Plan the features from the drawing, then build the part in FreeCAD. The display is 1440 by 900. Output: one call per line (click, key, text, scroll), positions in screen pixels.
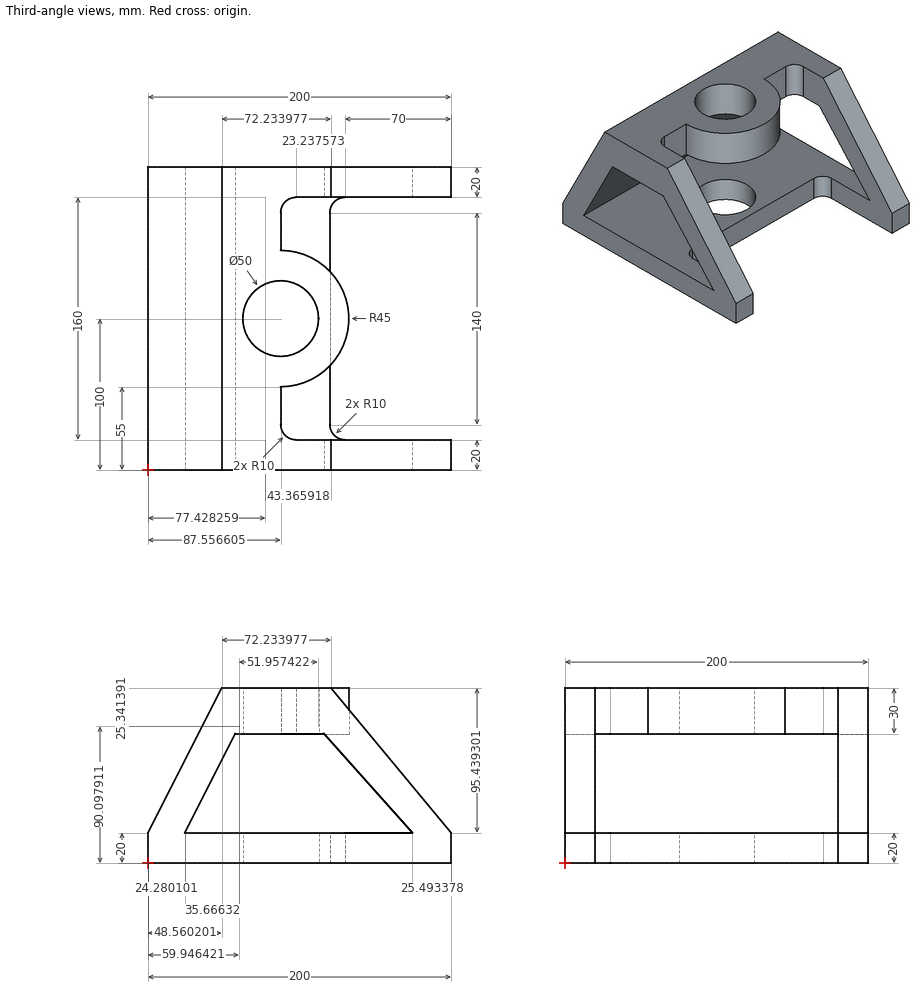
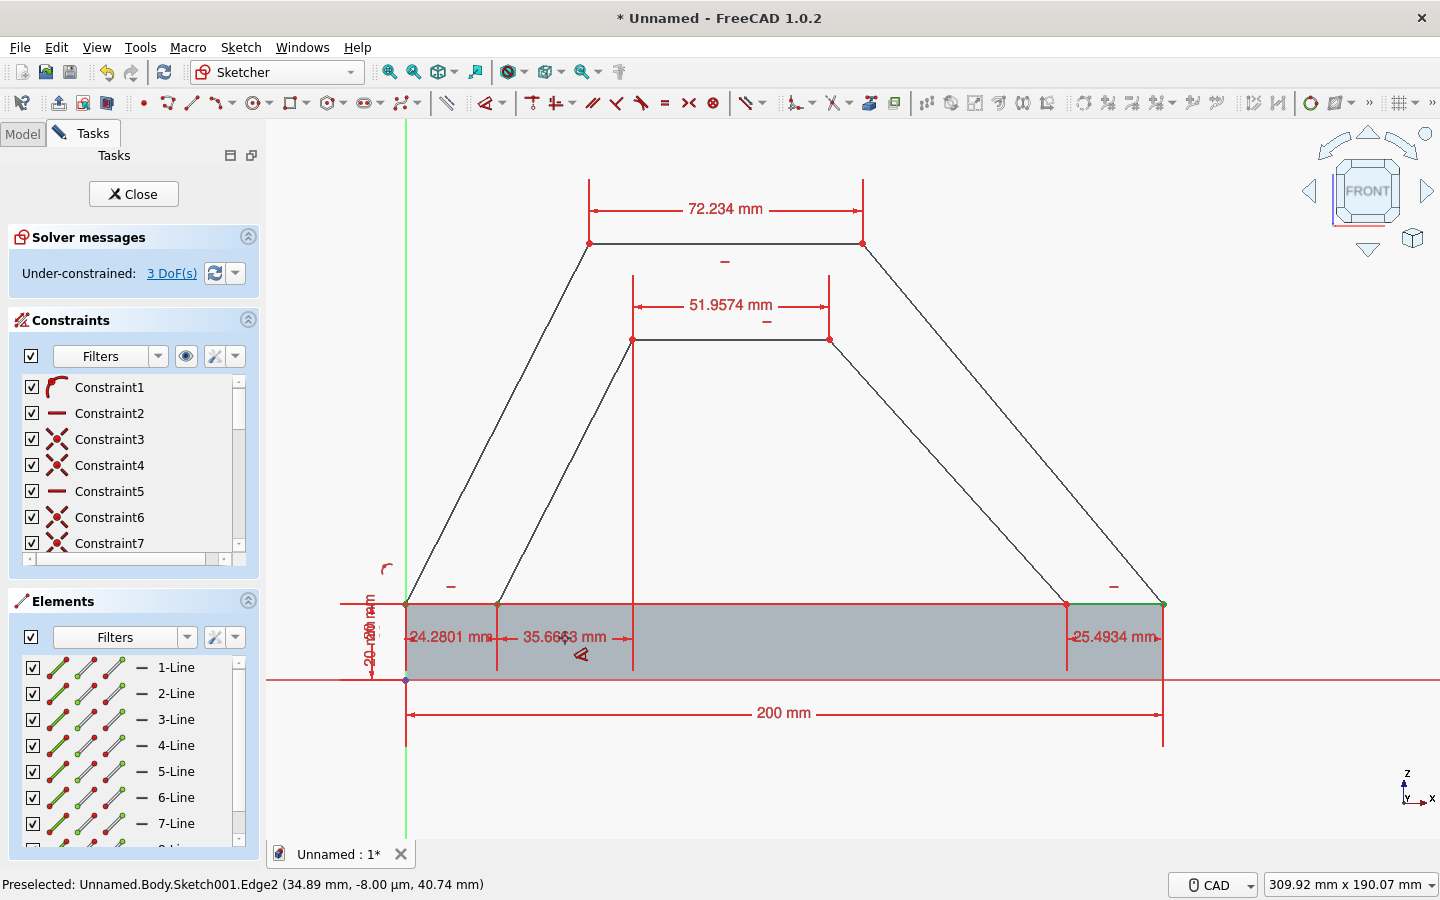
click(633, 340)
click(372, 510)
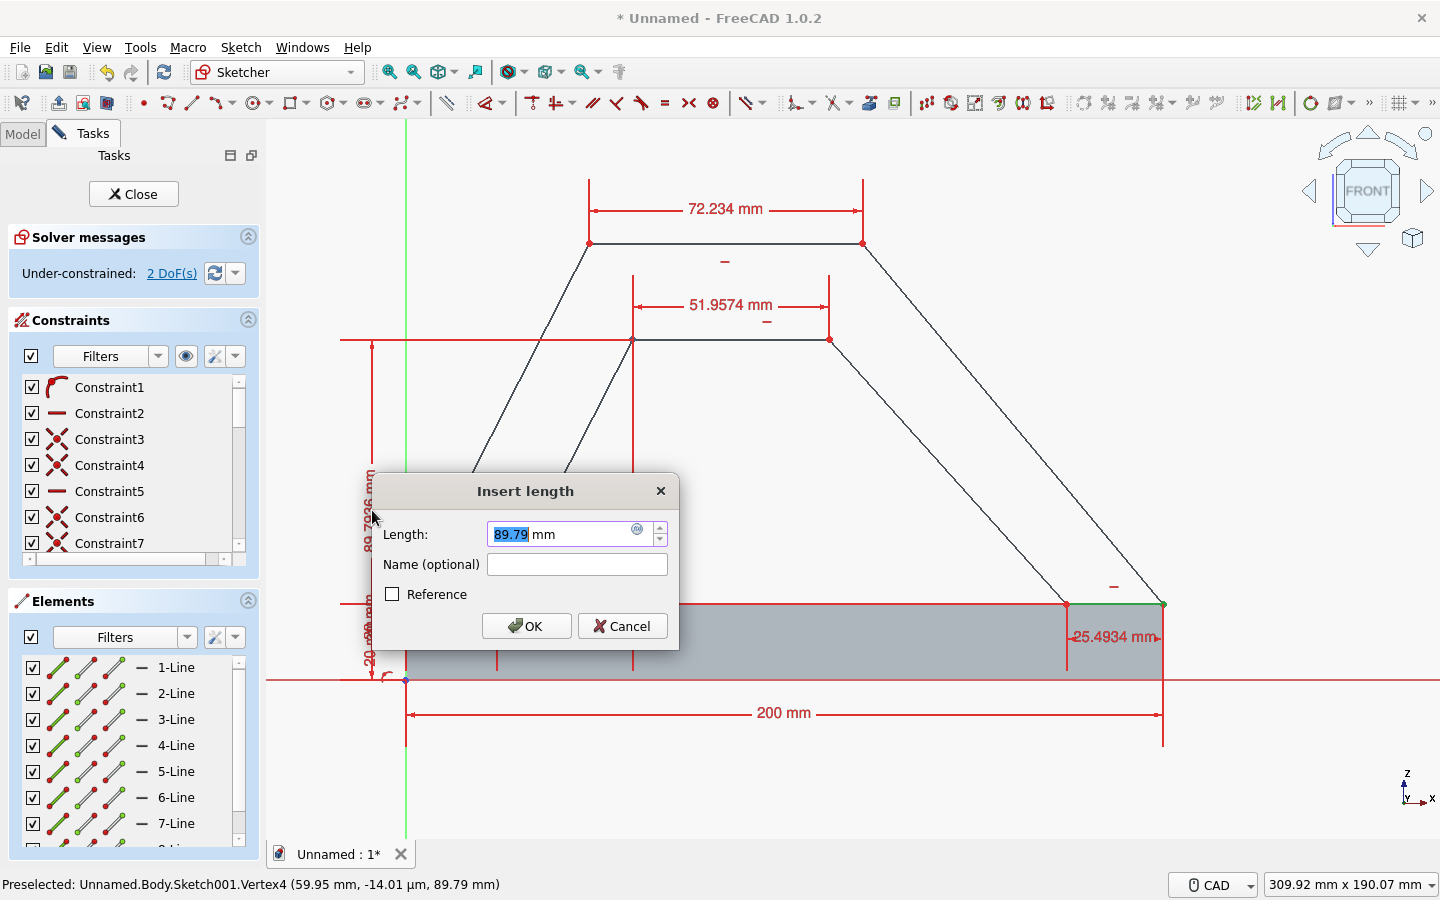
text(90.097911)
key(Return)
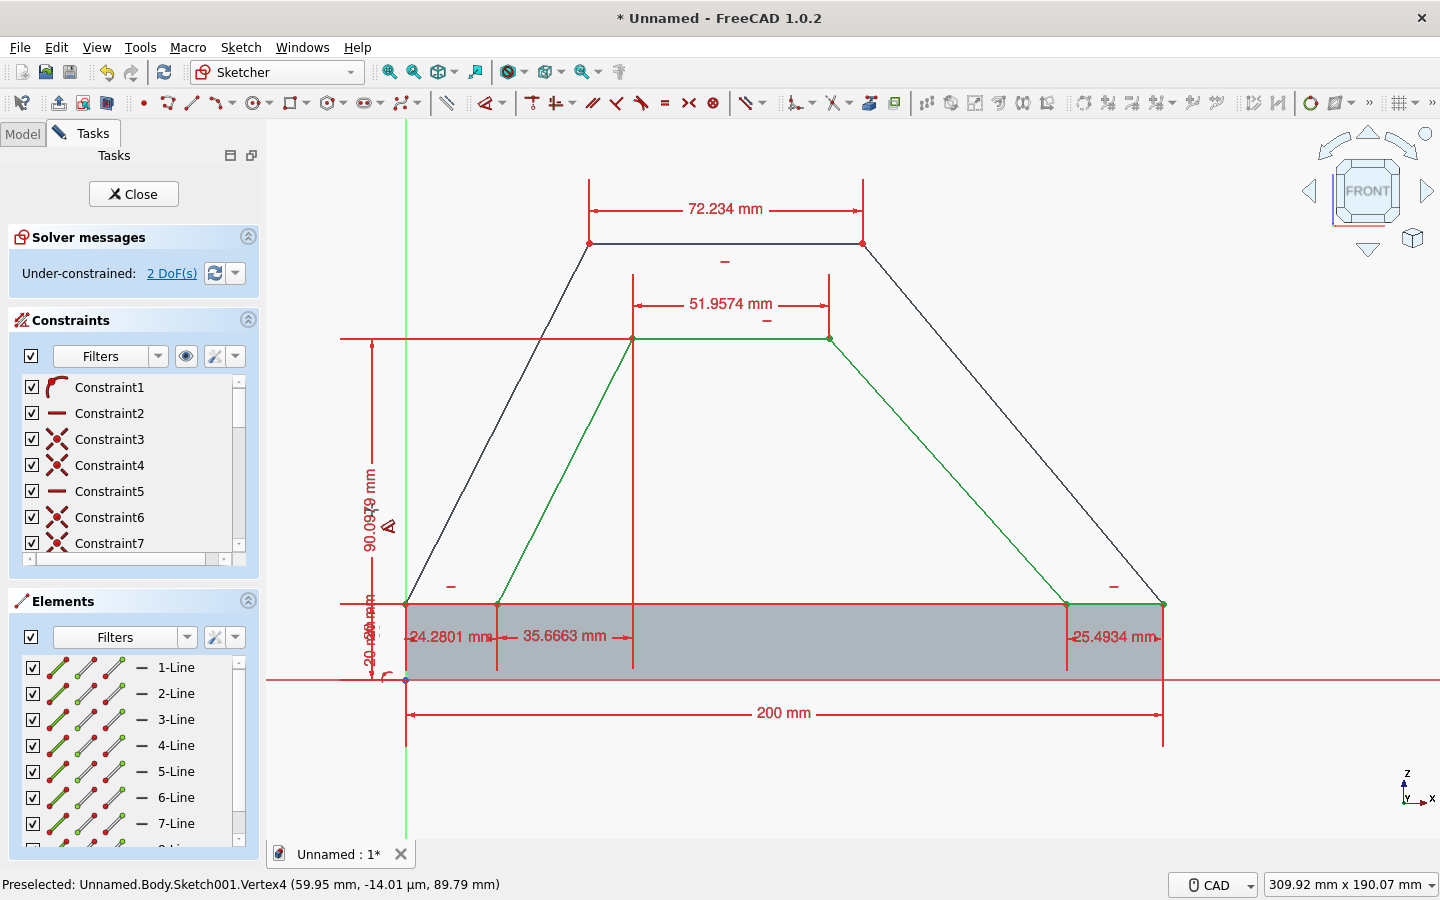
click(589, 244)
click(497, 714)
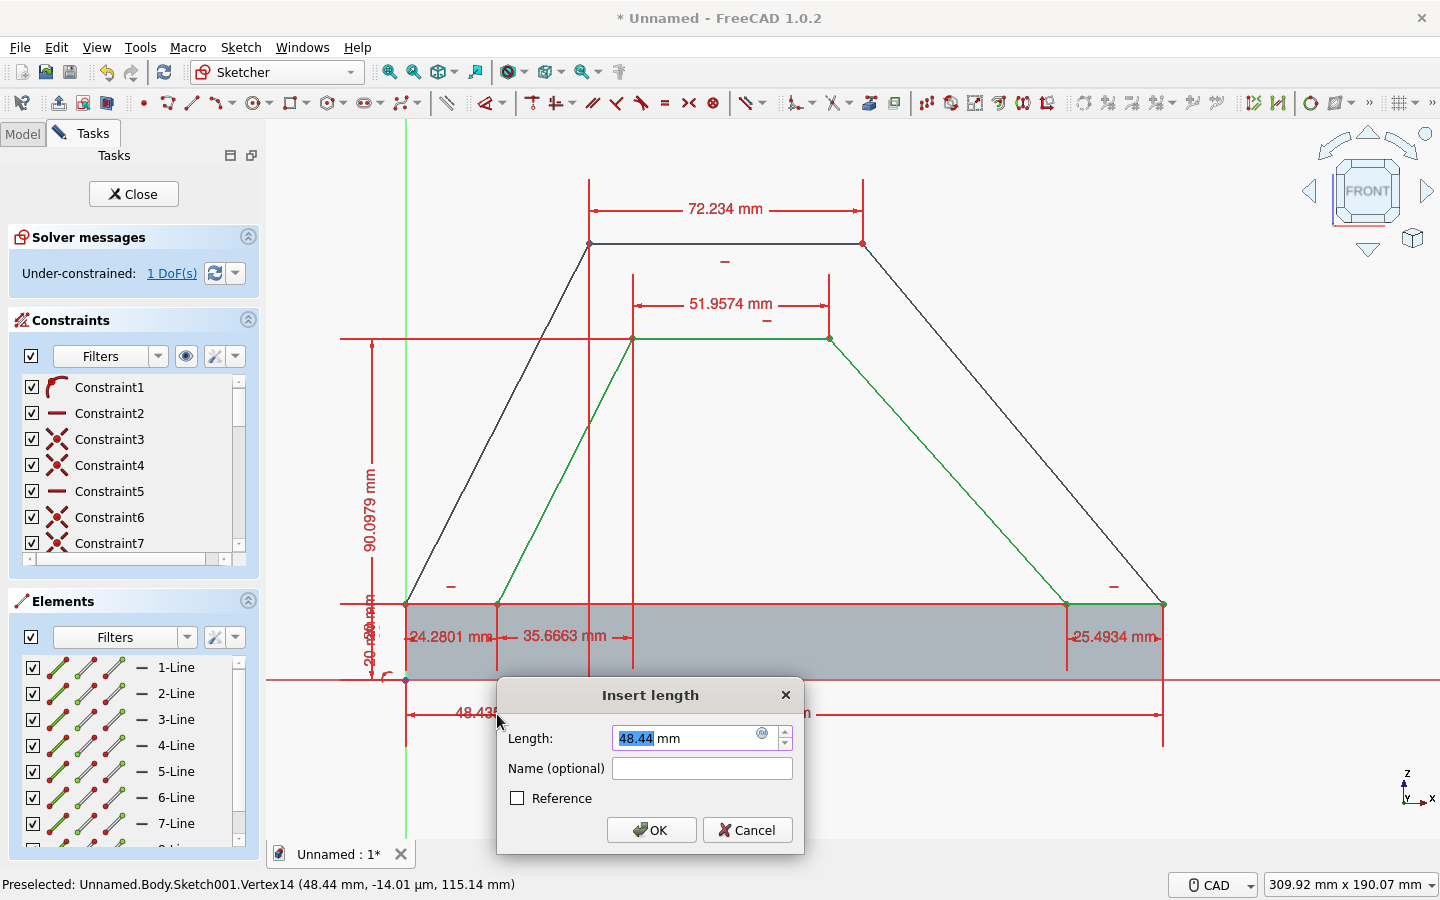
text(48.560201)
key(Return)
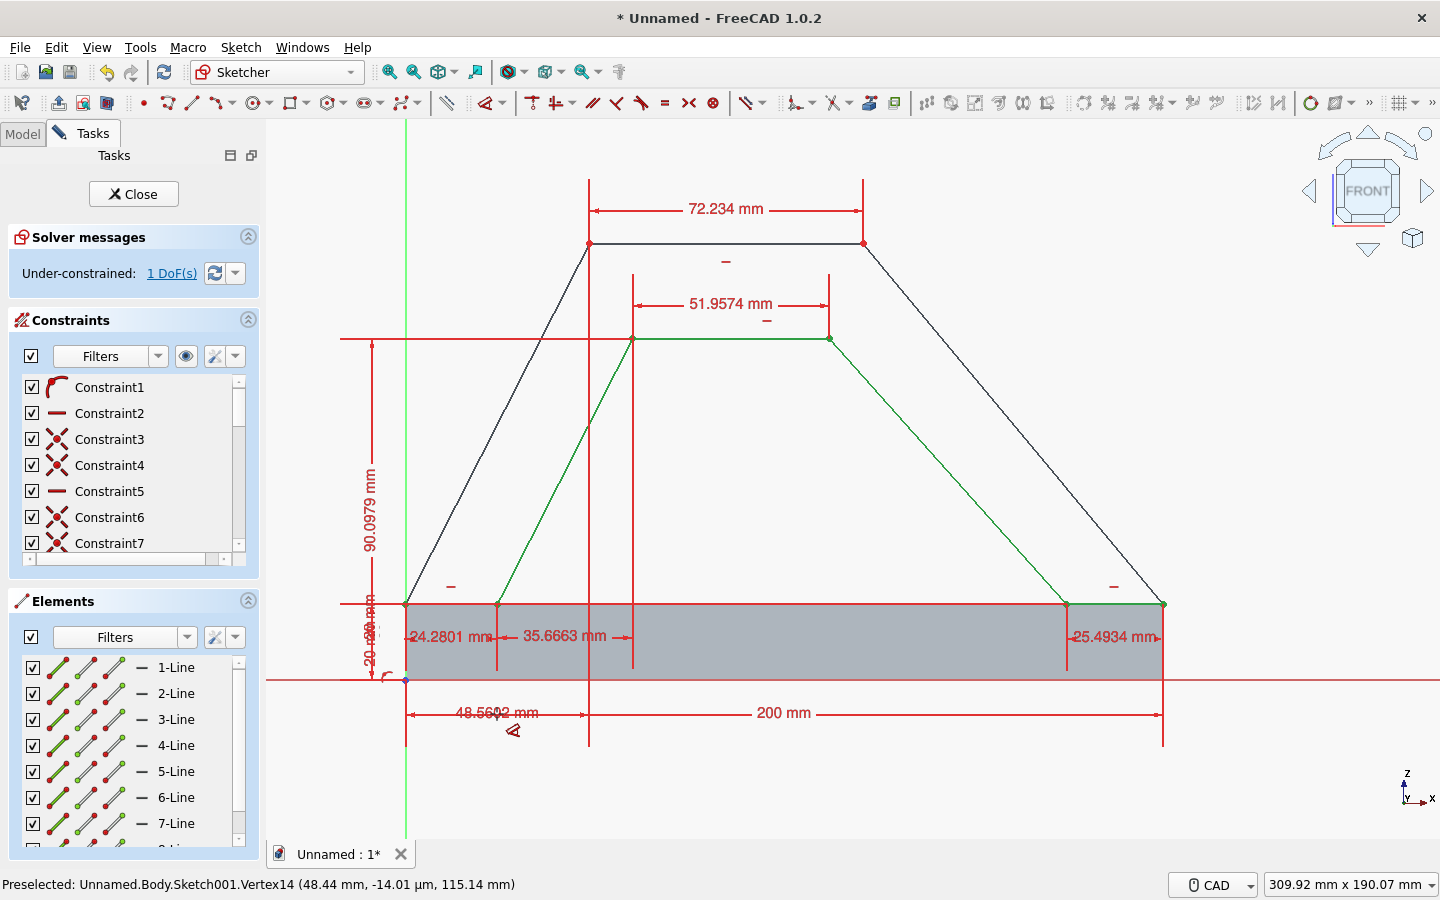
click(1073, 496)
click(1197, 424)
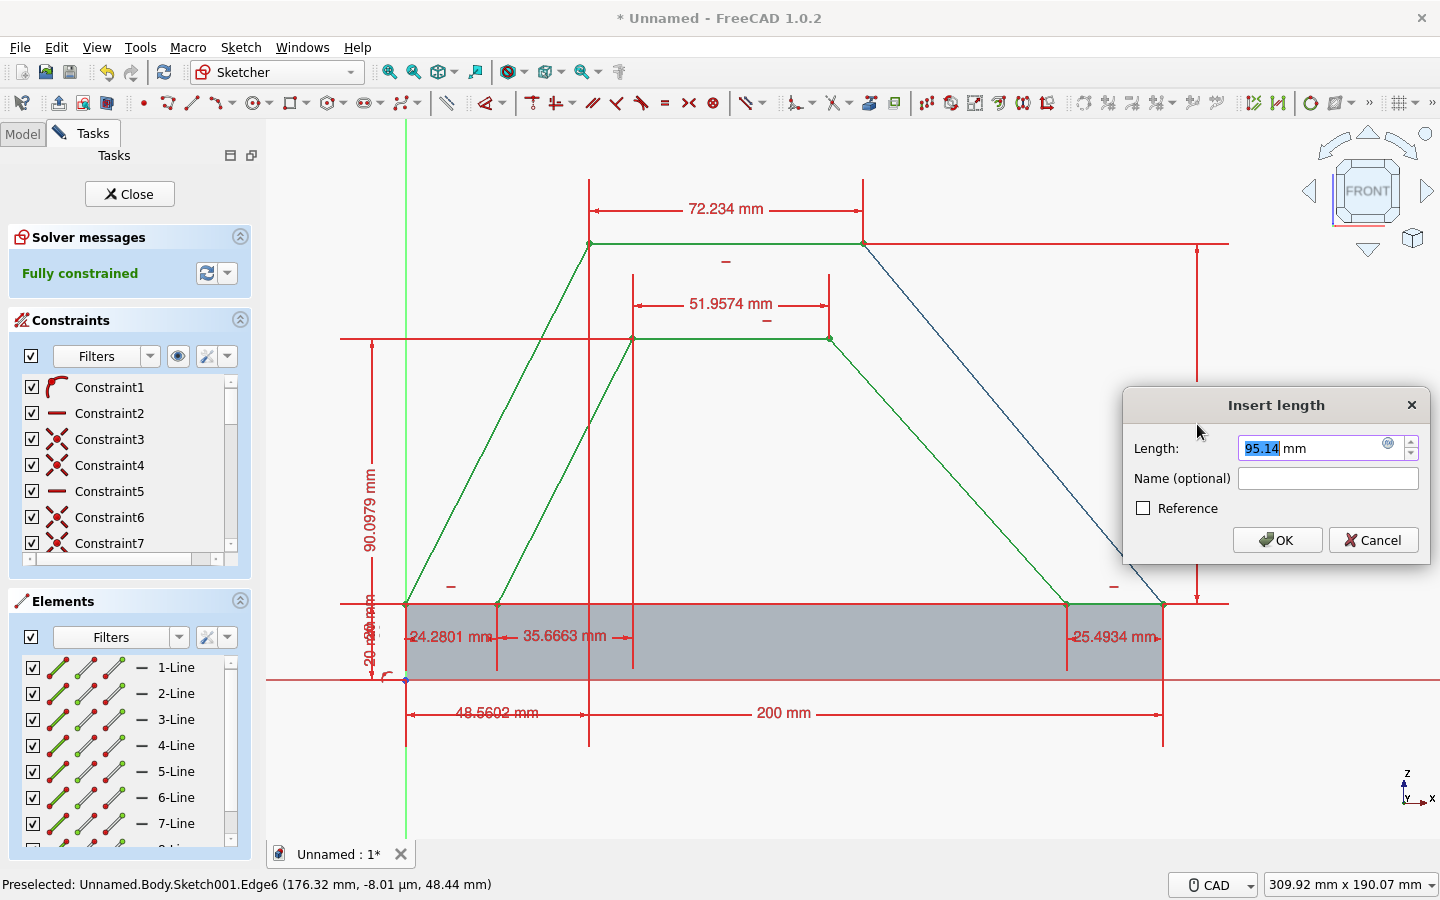
text(95.439301)
key(Return)
key(Escape)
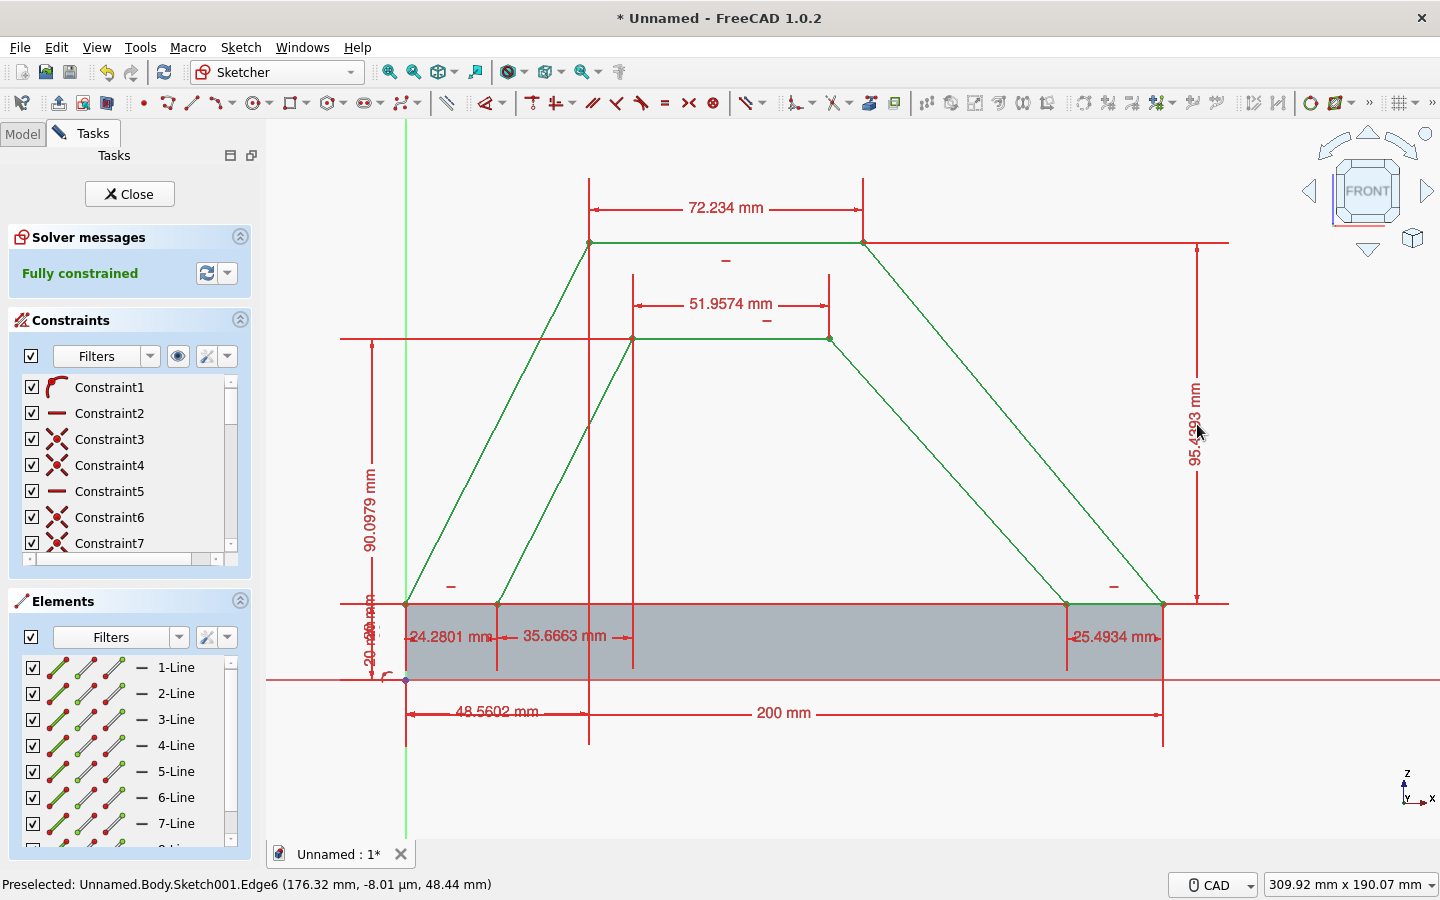
click(130, 194)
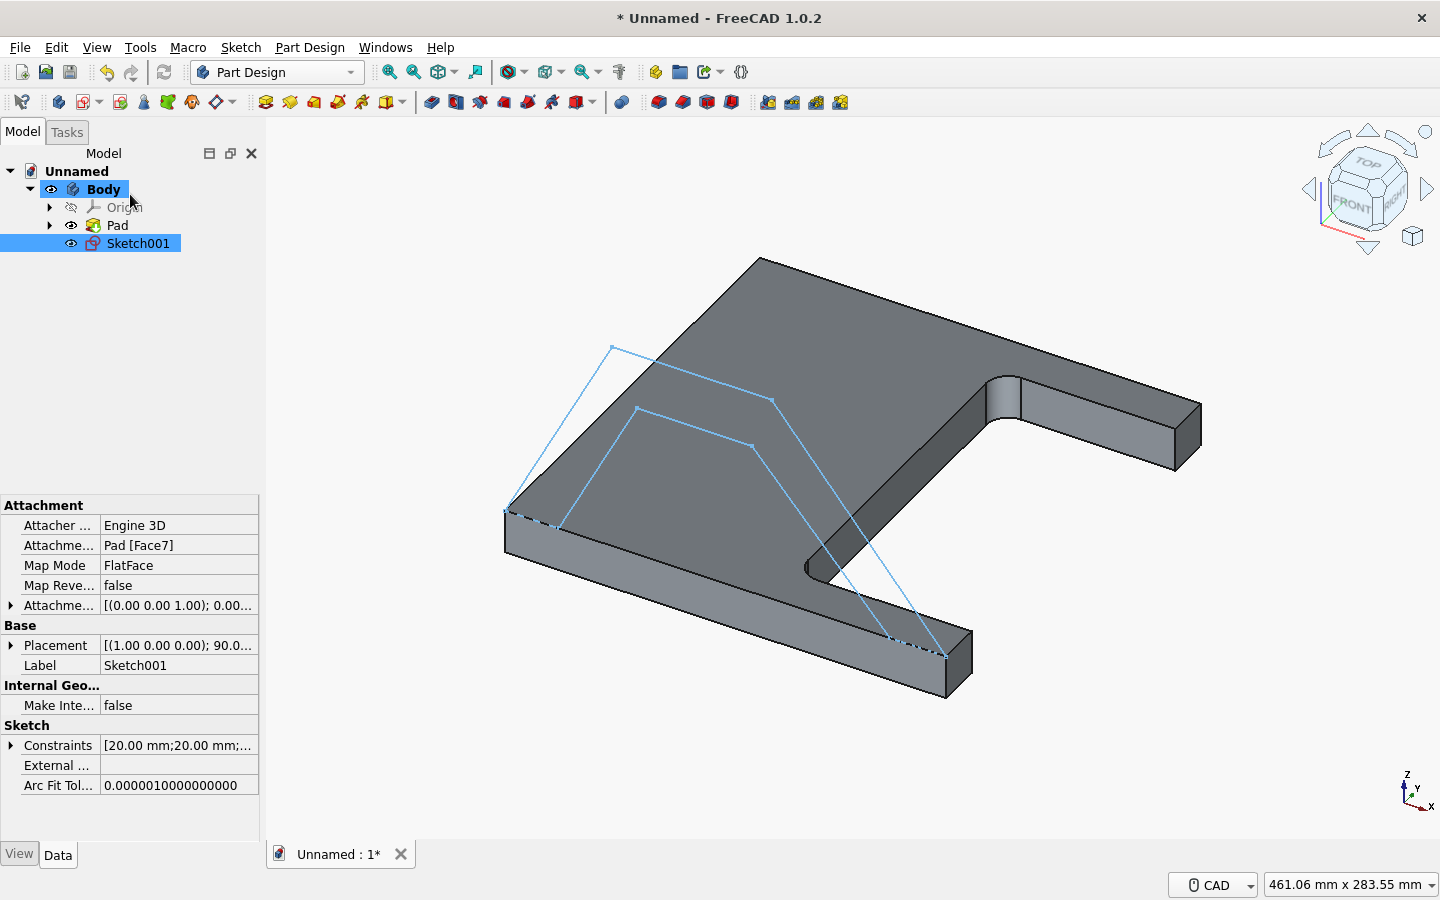
click(266, 102)